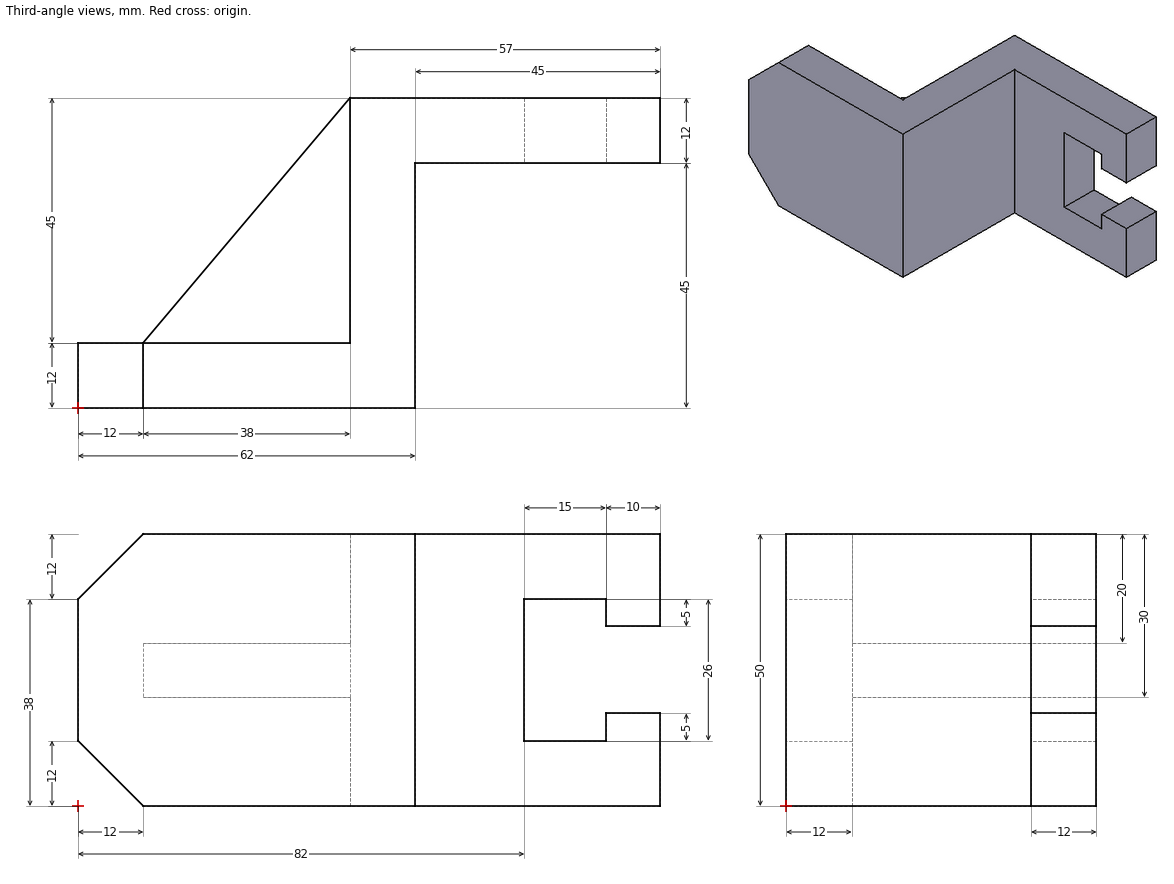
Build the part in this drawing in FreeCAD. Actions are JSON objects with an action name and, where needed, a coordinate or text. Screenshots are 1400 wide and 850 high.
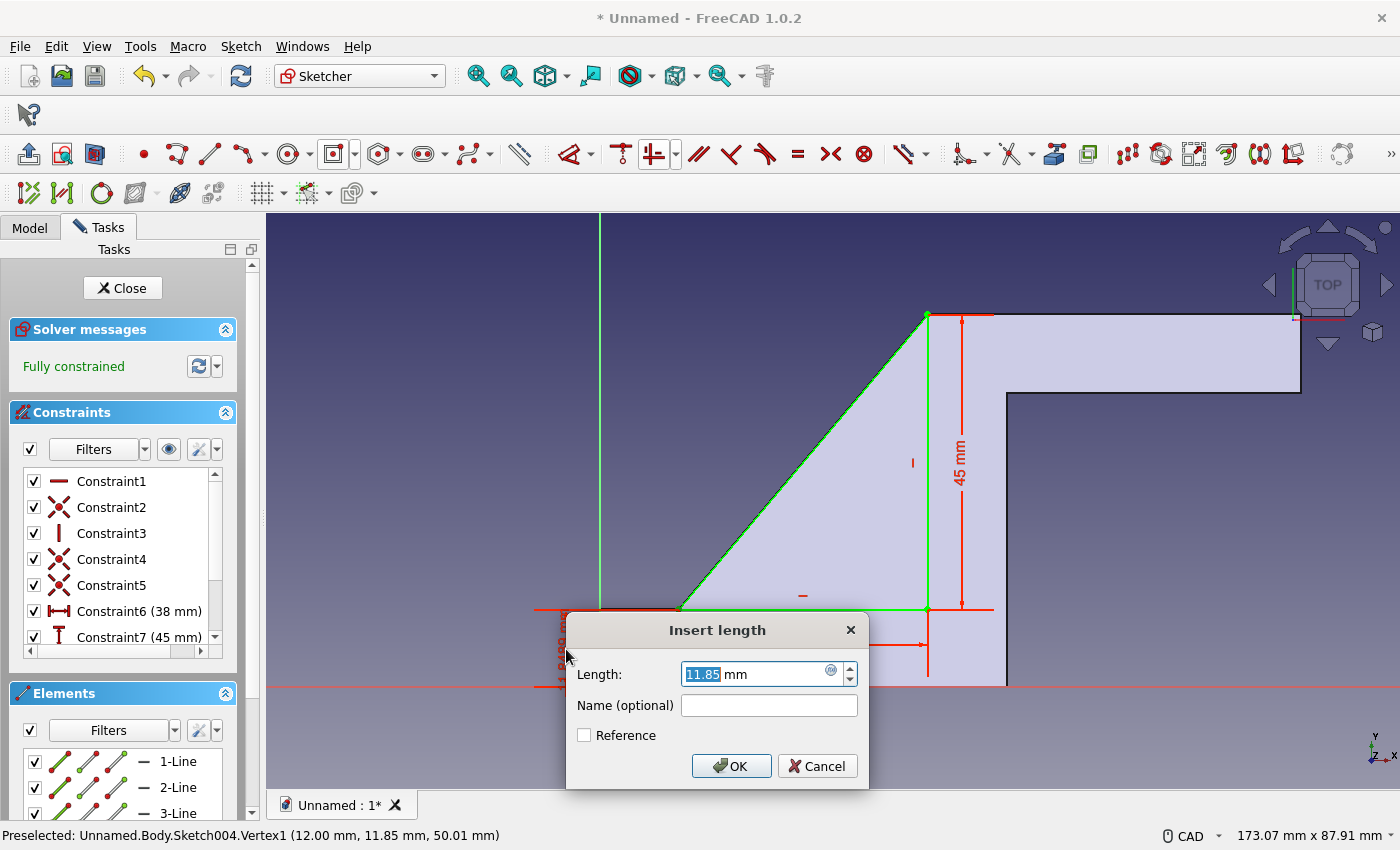
{"action": "type", "text": "12"}
{"action": "key", "text": "Return"}
{"action": "key", "text": "Escape"}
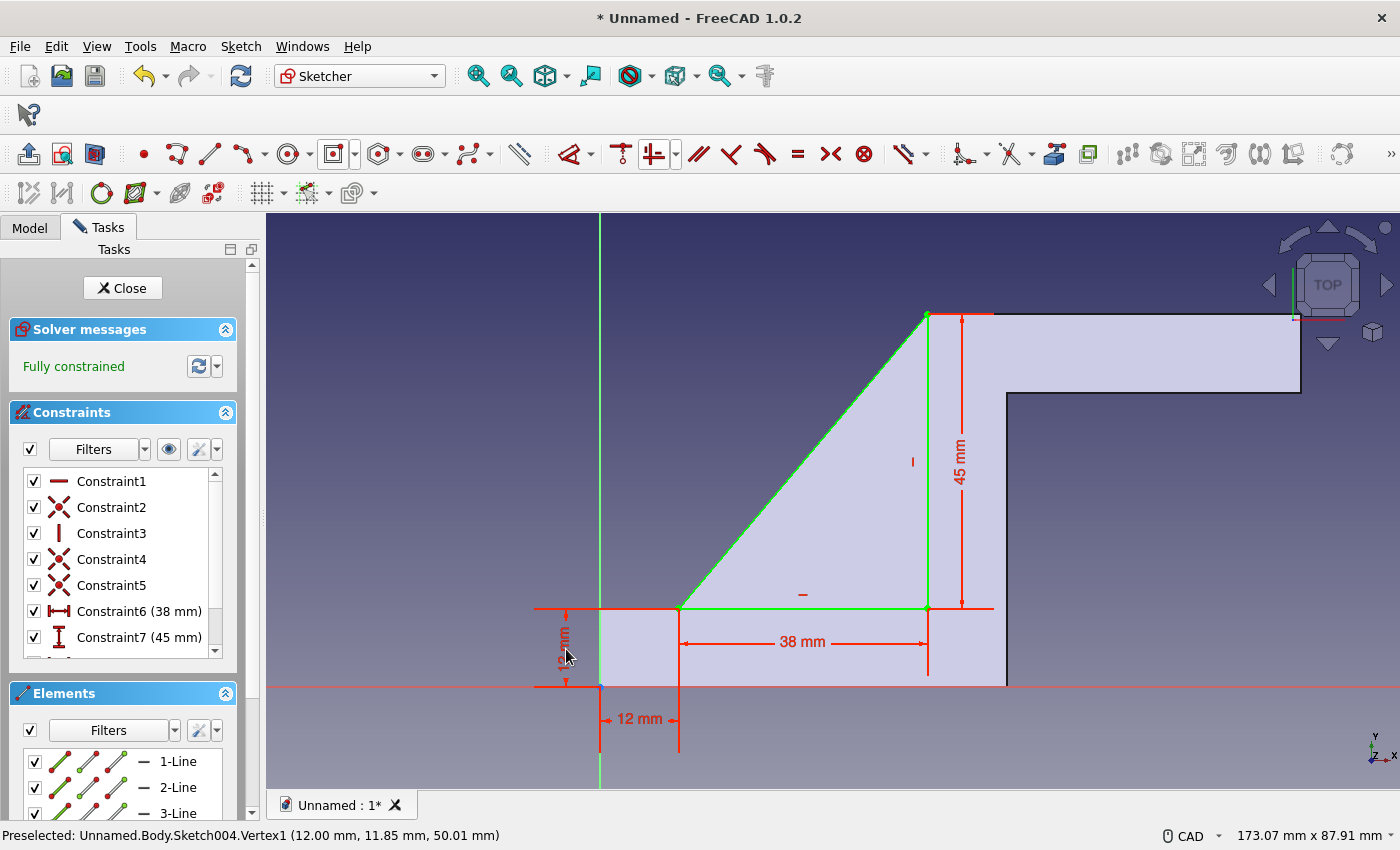
{"action": "left_click", "coordinate": [123, 288]}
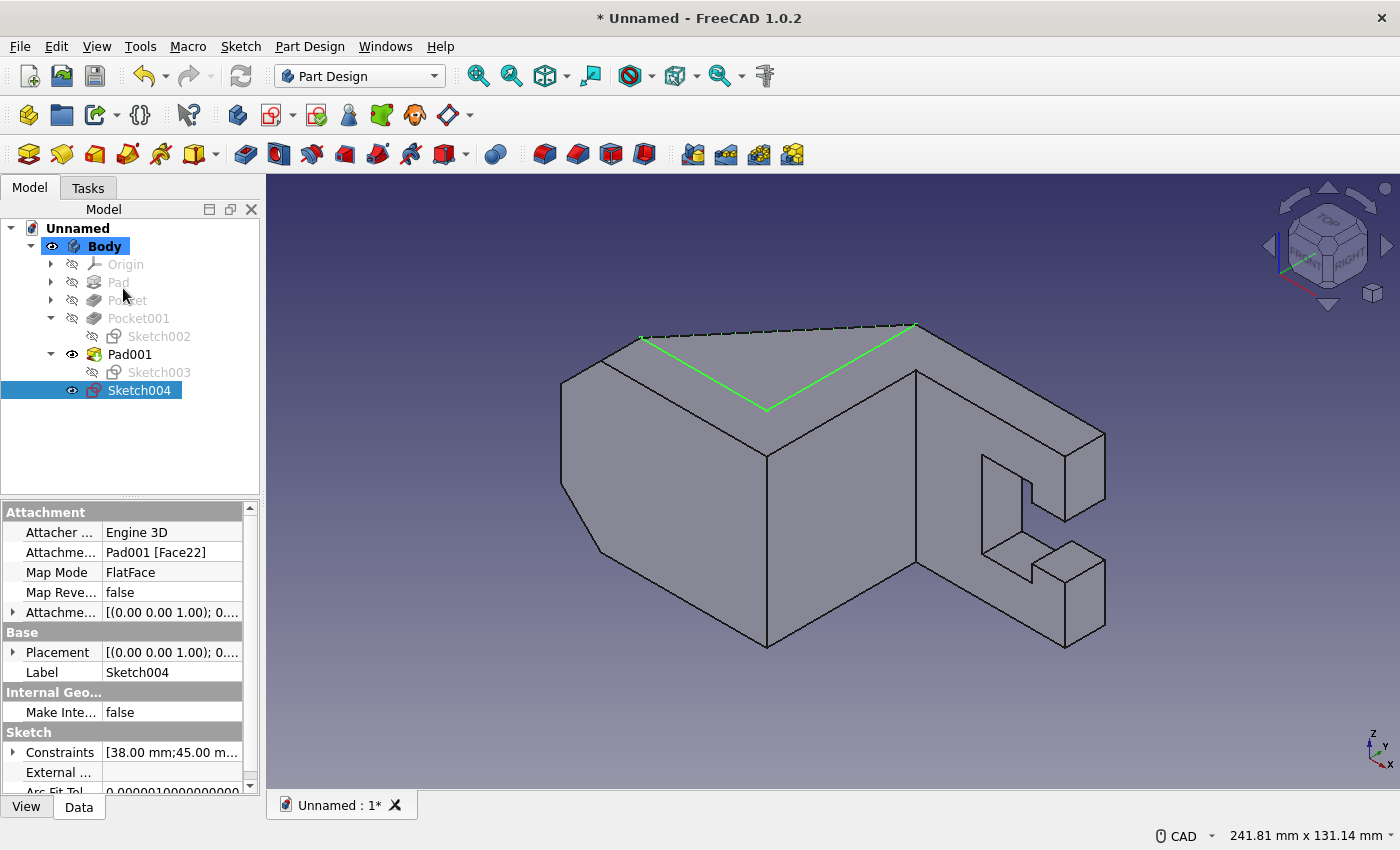
{"action": "left_click", "coordinate": [246, 154]}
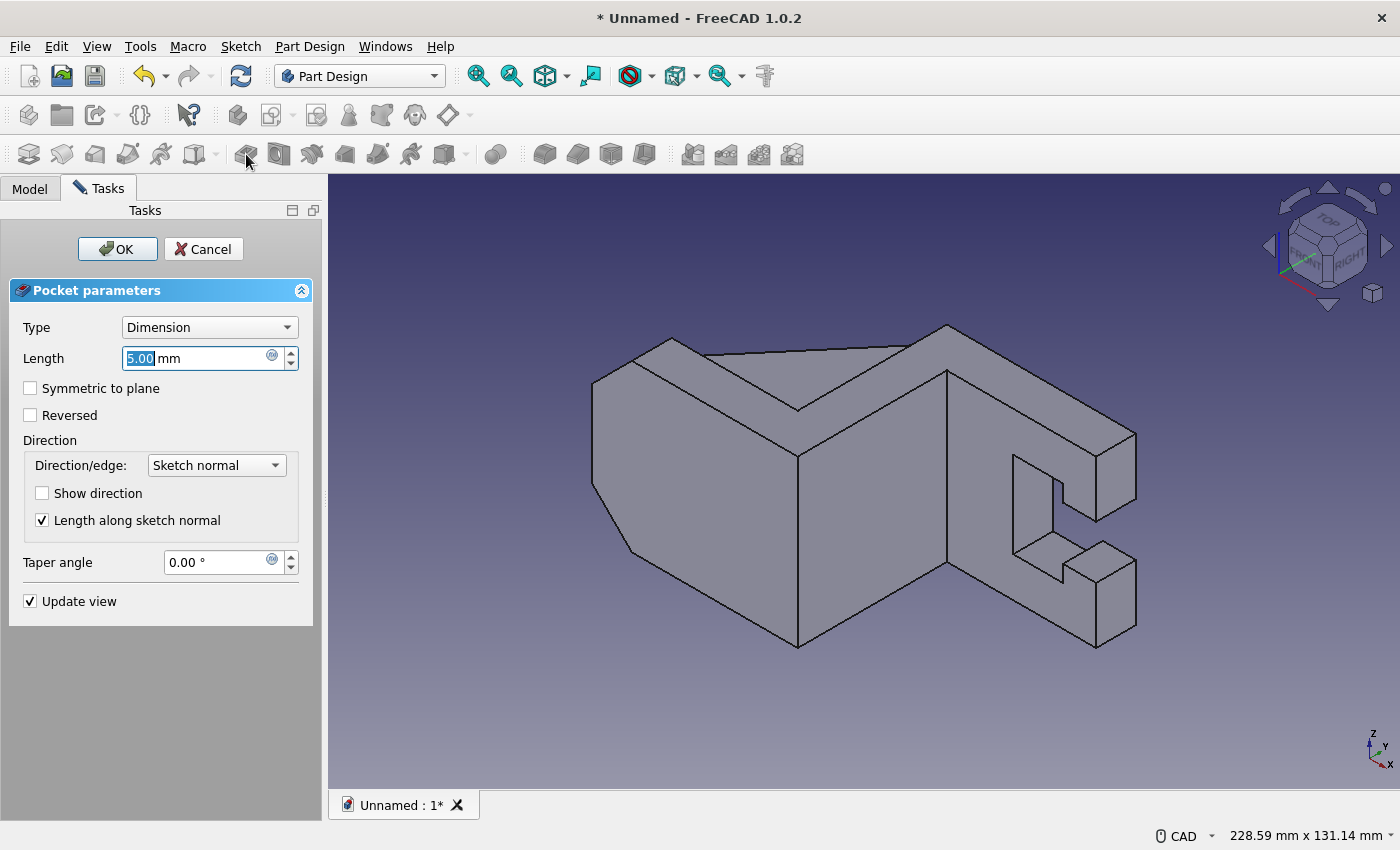
{"action": "type", "text": "20"}
{"action": "key", "text": "Tab"}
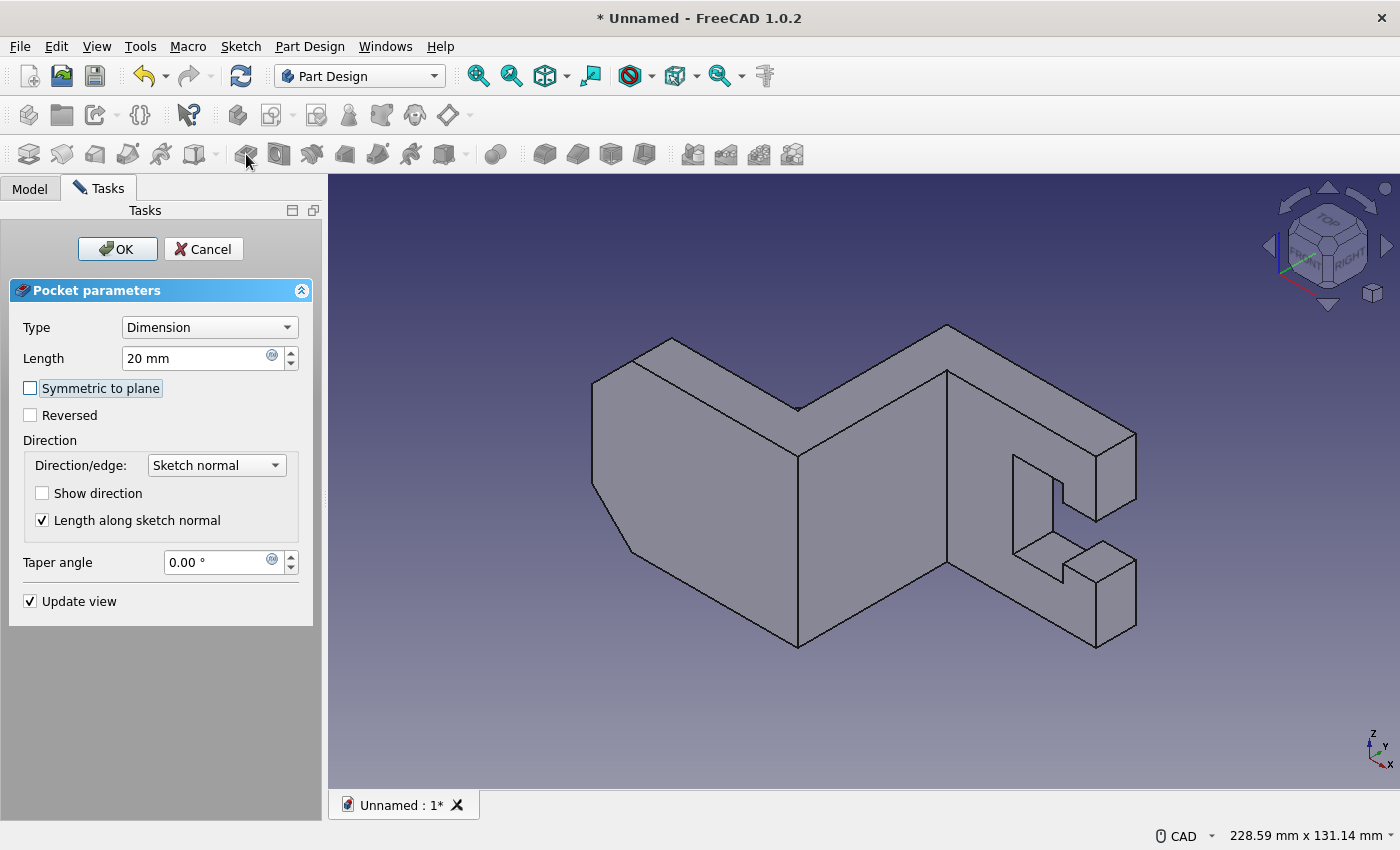
{"action": "left_click", "coordinate": [118, 249]}